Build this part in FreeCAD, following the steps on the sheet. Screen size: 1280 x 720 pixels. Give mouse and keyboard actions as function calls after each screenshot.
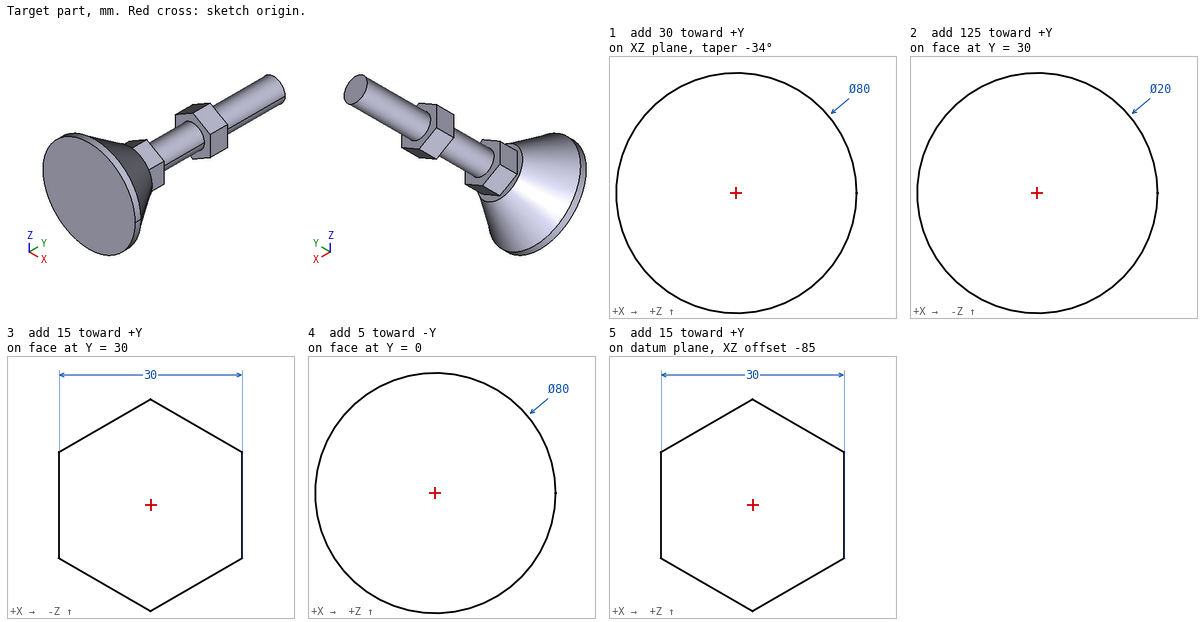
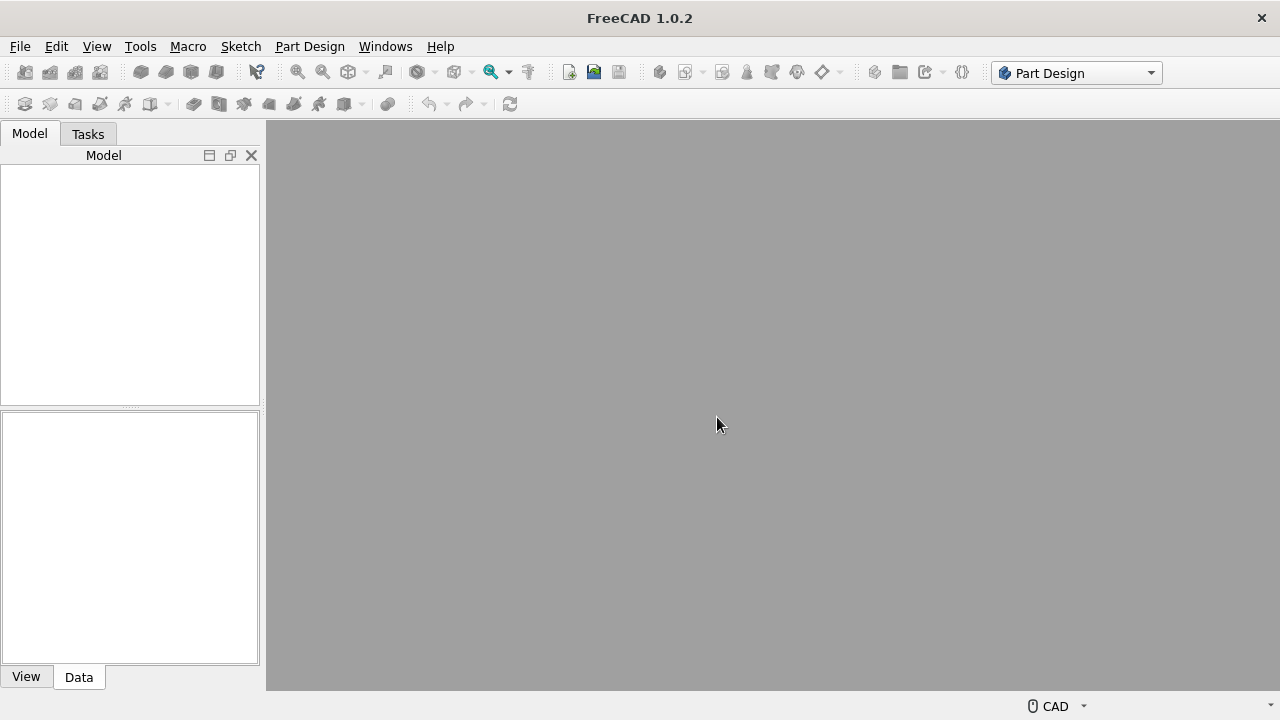
click(569, 72)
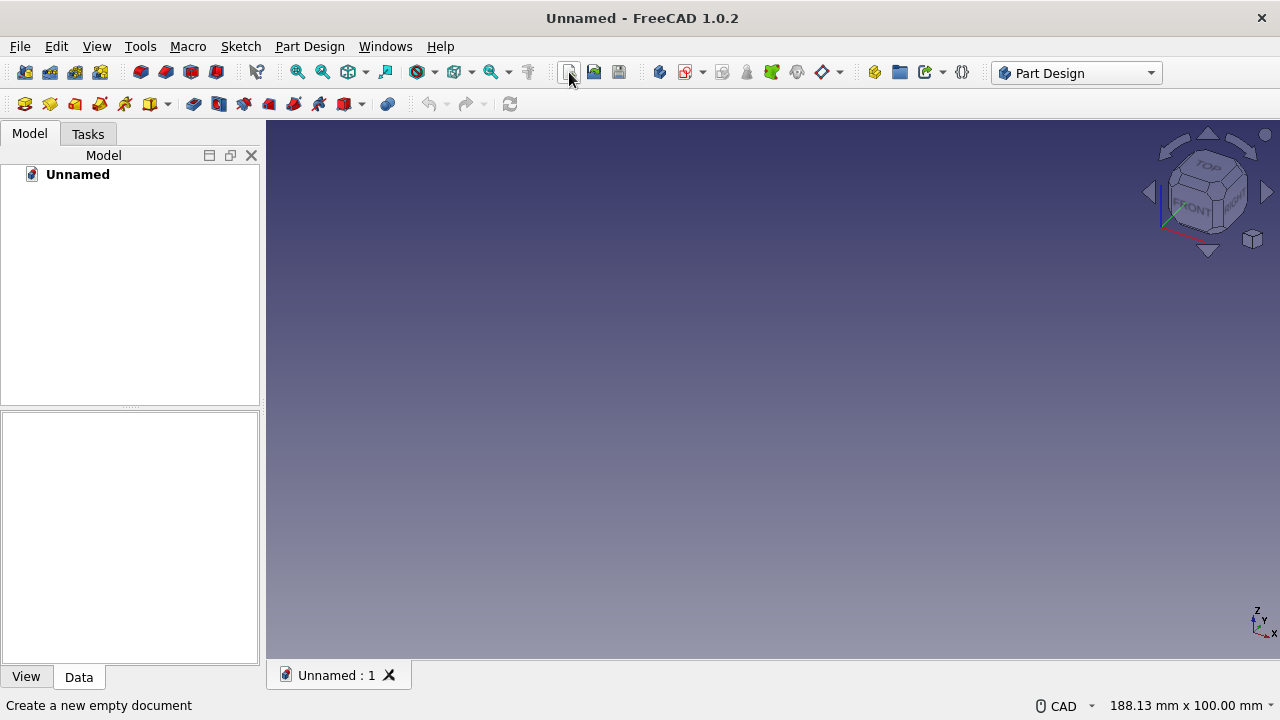
click(684, 72)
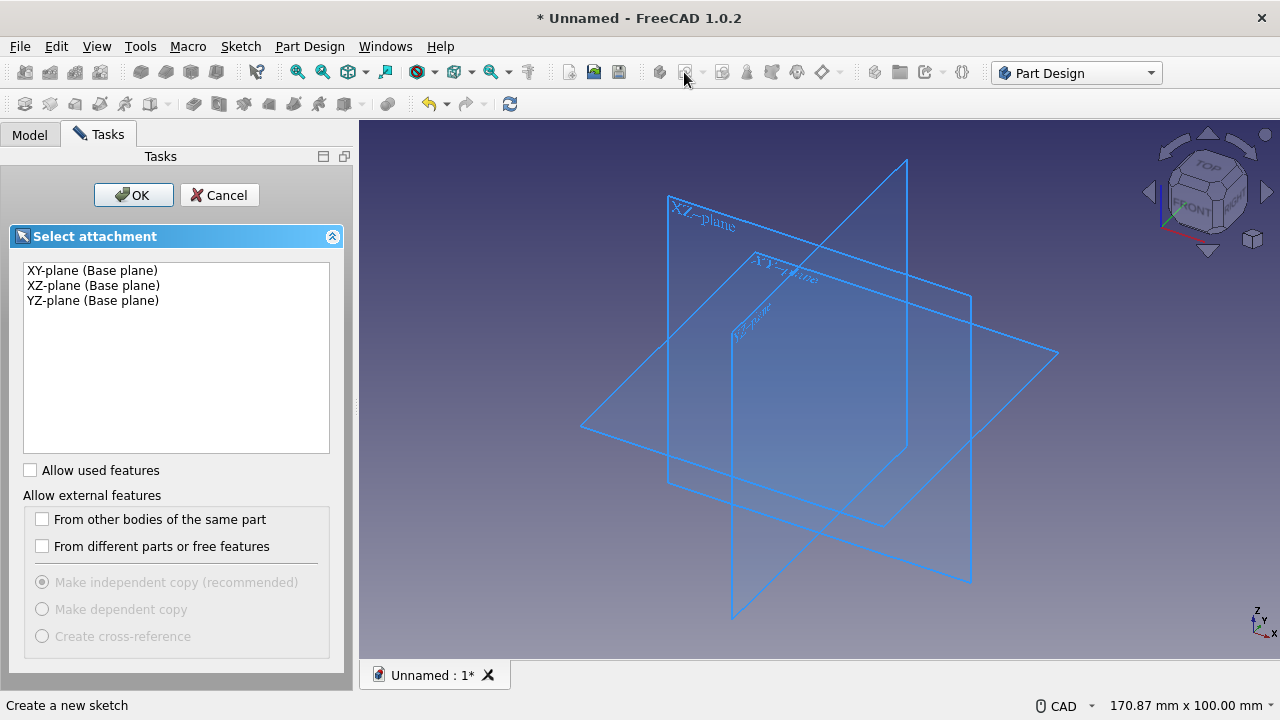
click(84, 286)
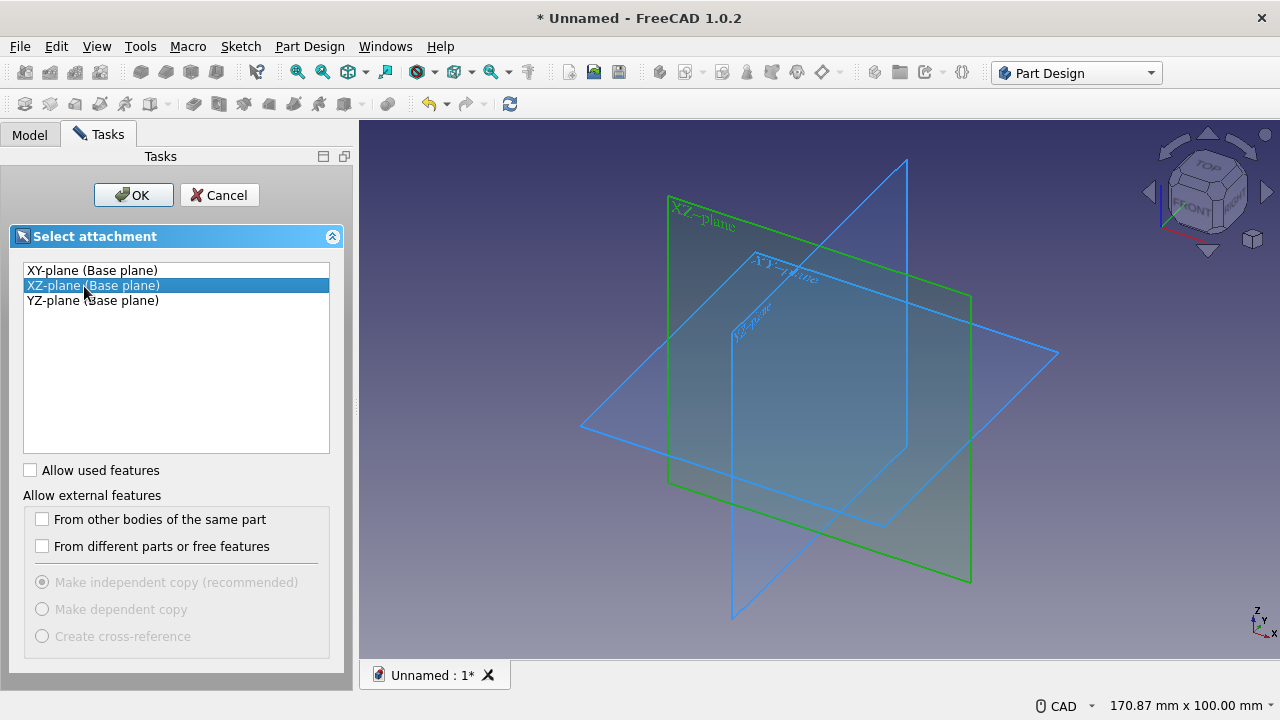
click(134, 195)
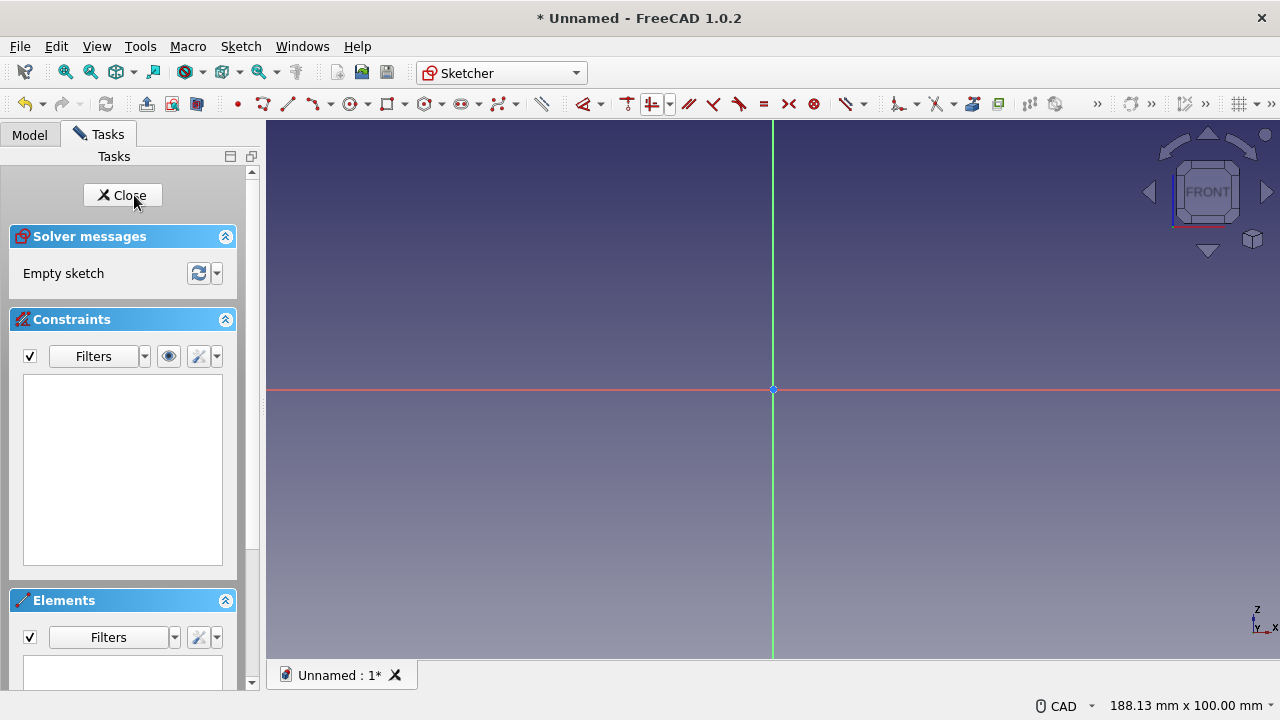
click(350, 104)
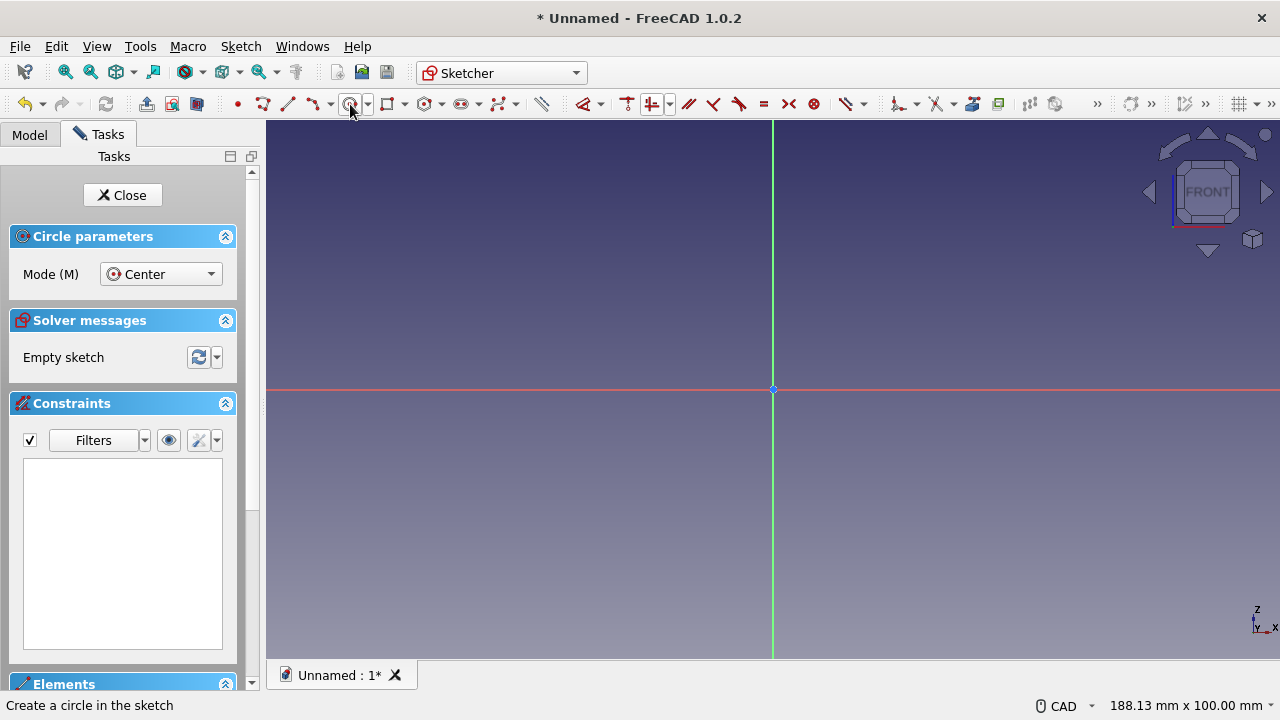
click(773, 390)
move(925, 237)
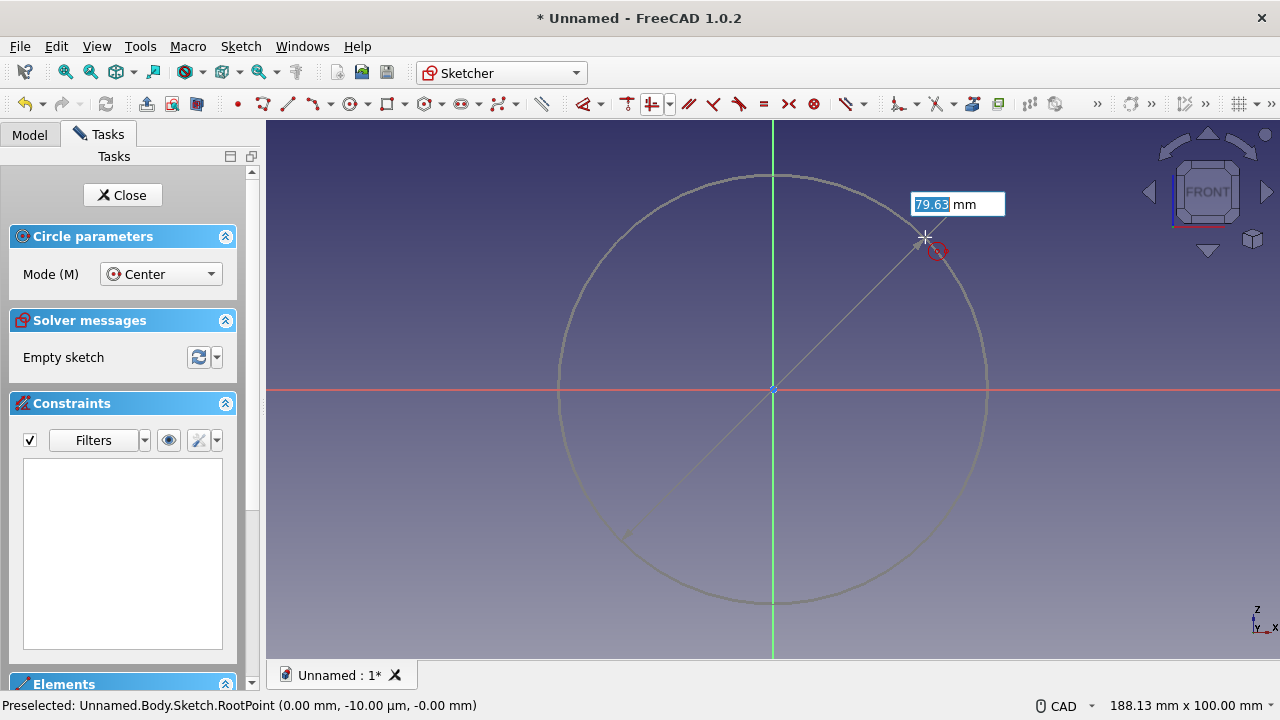
text(80)
key(Return)
key(Escape)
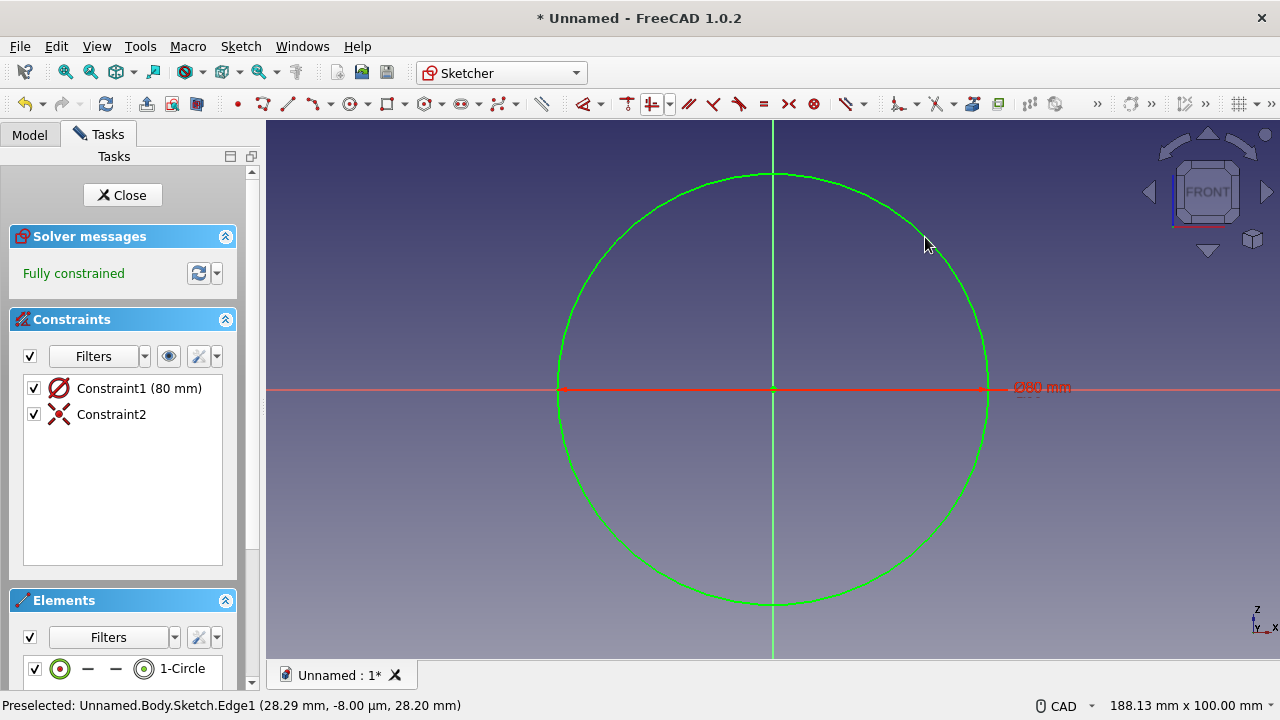
click(123, 195)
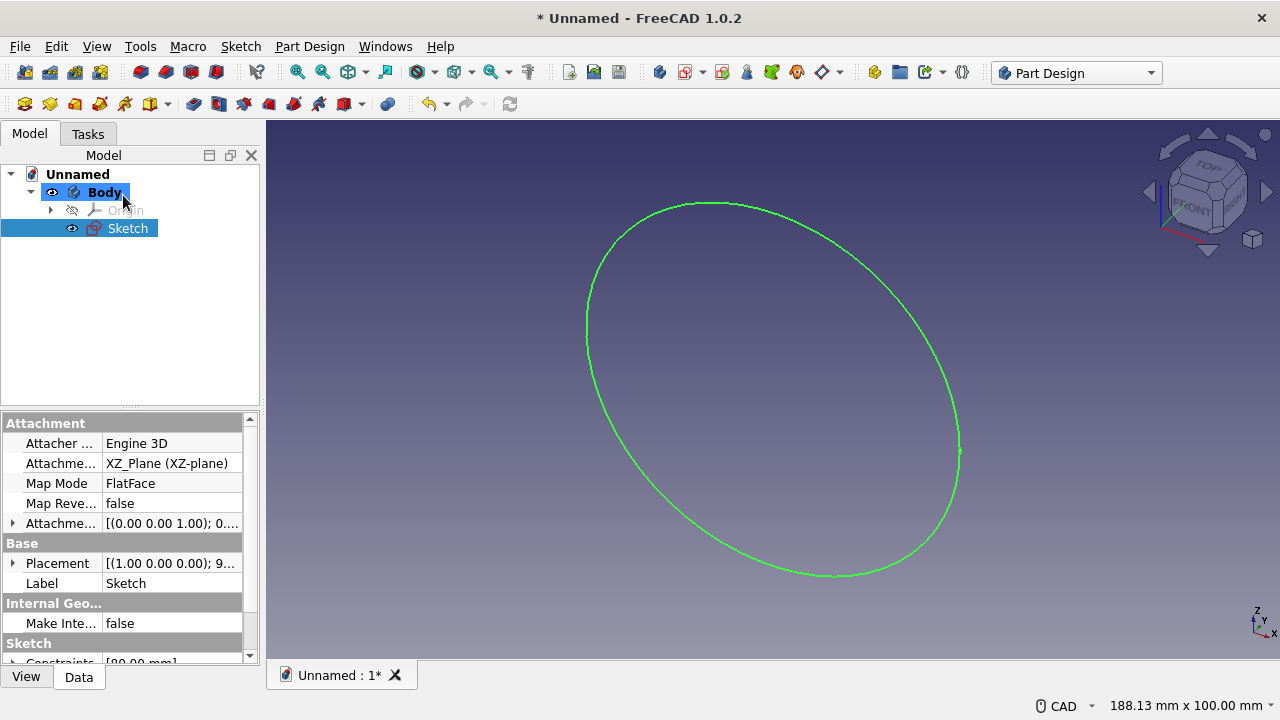
click(25, 104)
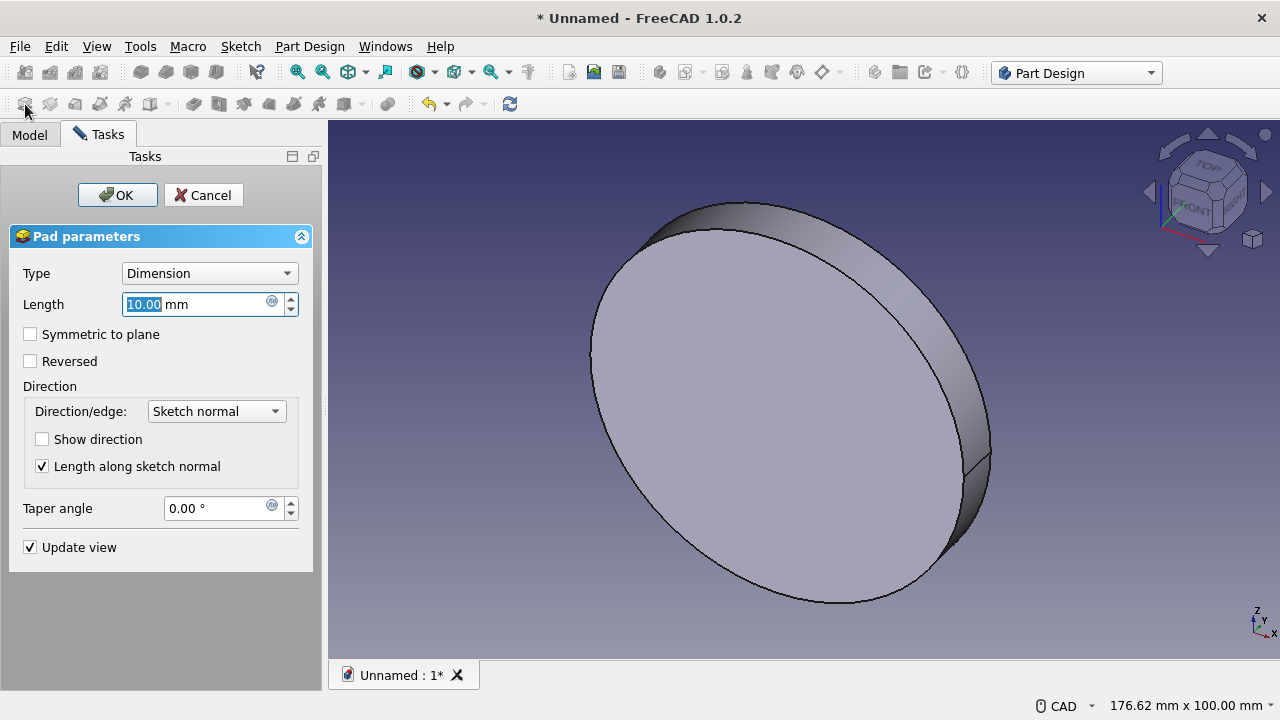
text(30)
key(Tab)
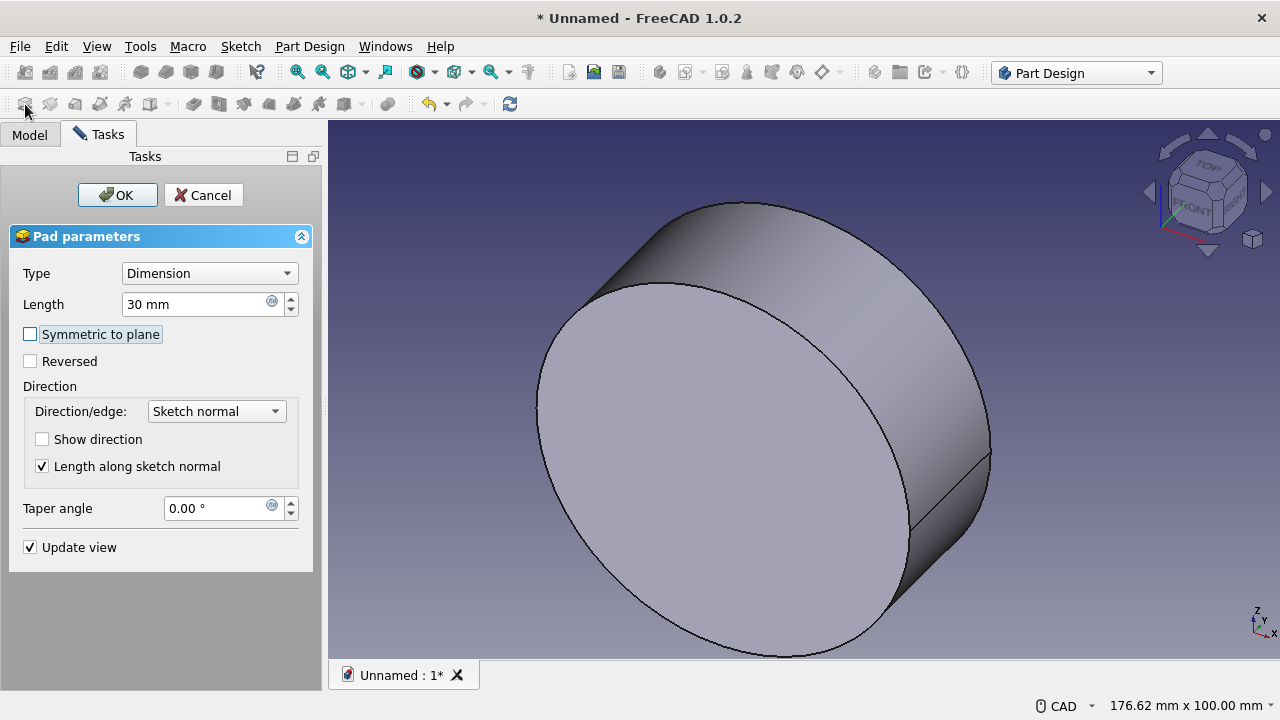
click(31, 361)